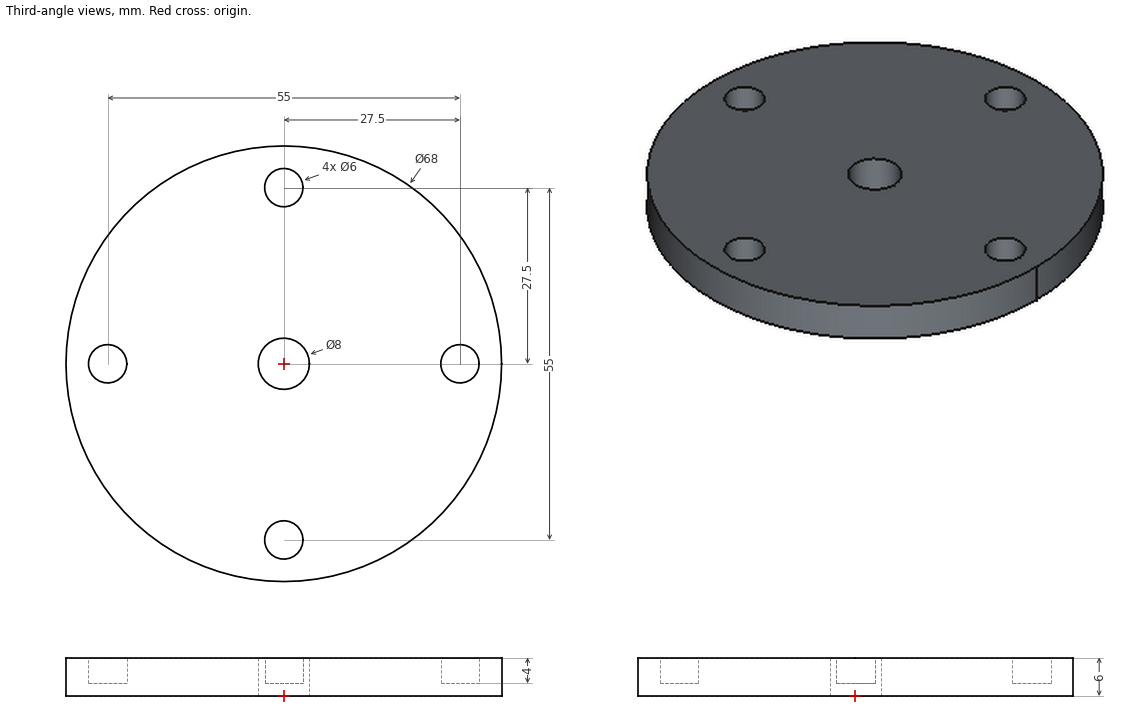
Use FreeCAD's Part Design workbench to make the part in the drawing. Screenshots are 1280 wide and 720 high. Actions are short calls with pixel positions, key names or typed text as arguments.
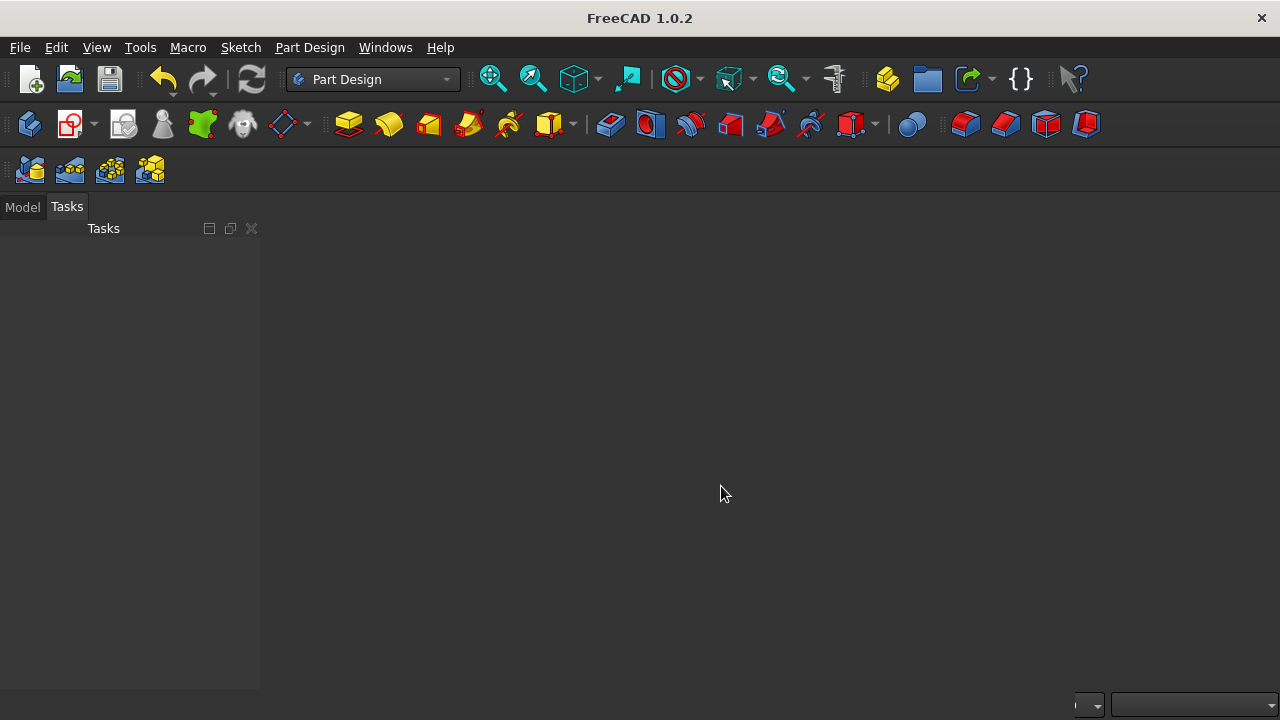
click(30, 80)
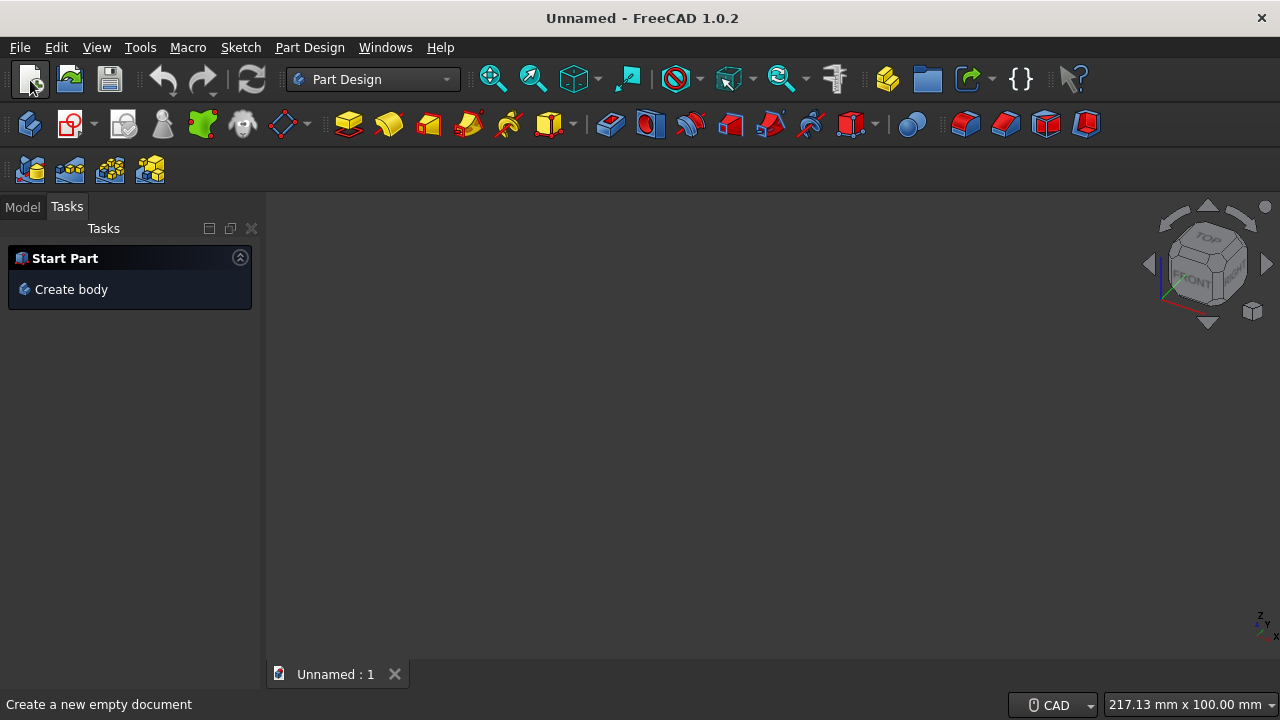
click(70, 124)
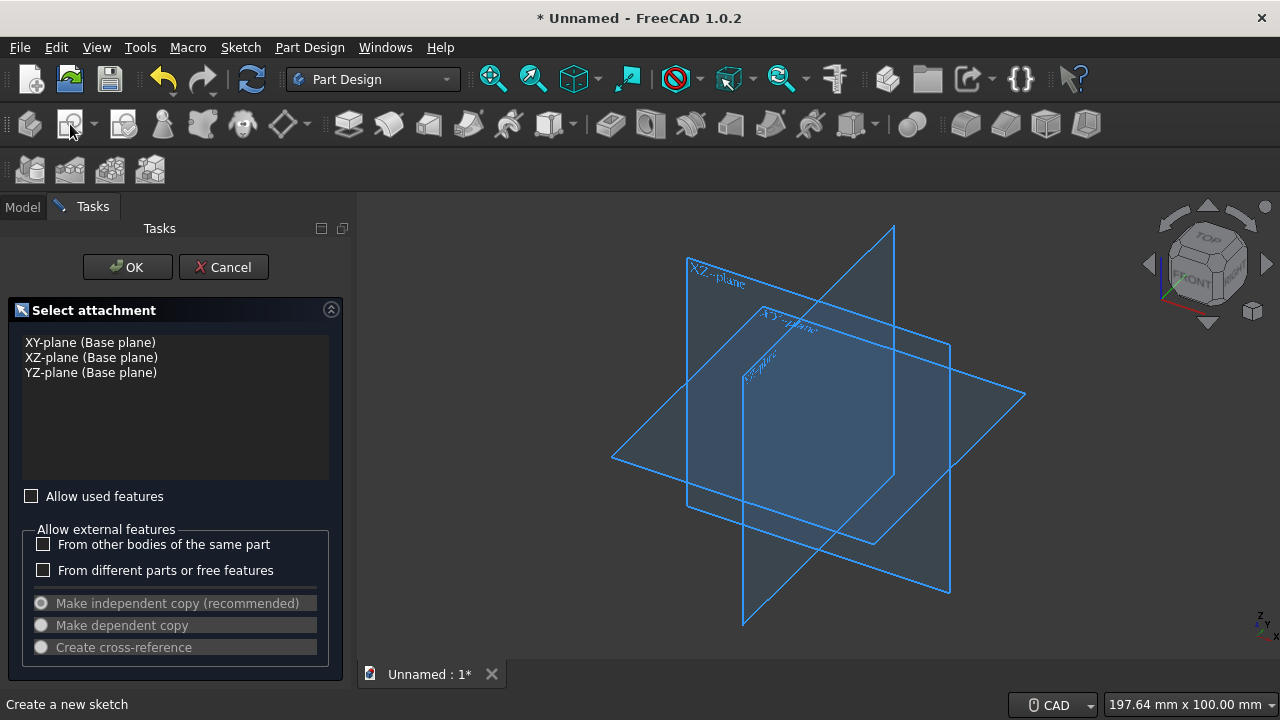
click(82, 342)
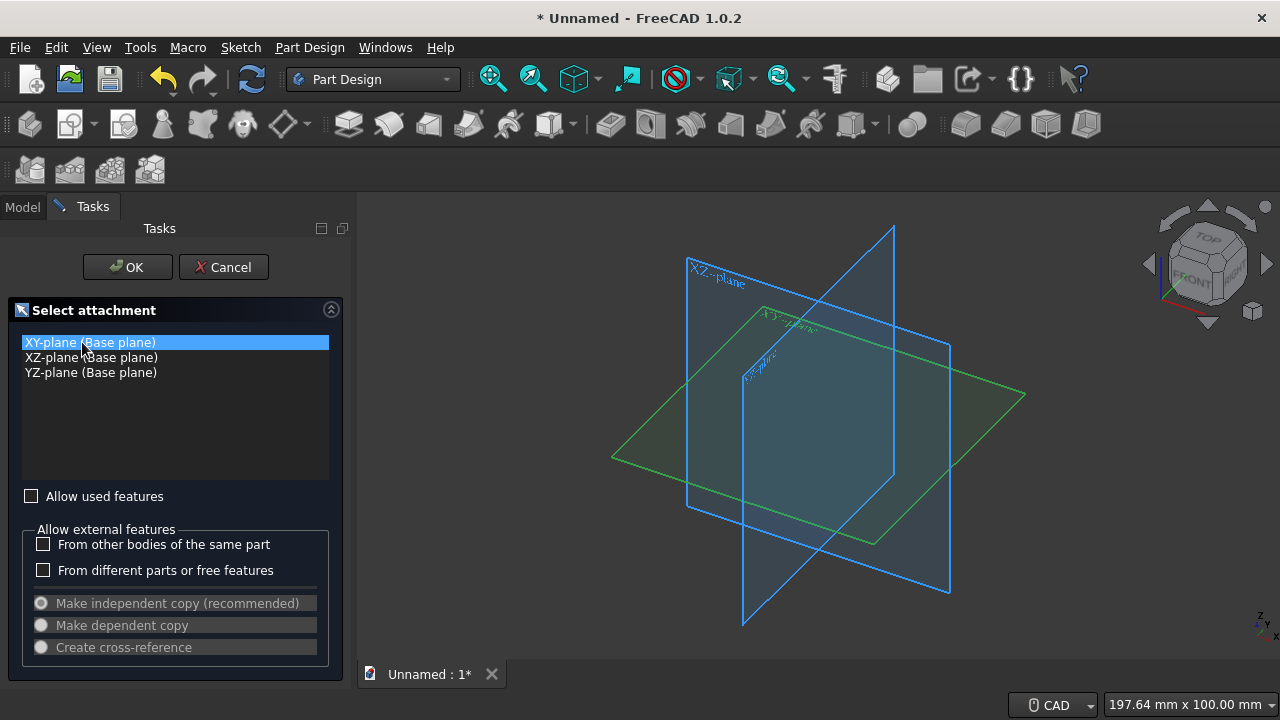
click(128, 267)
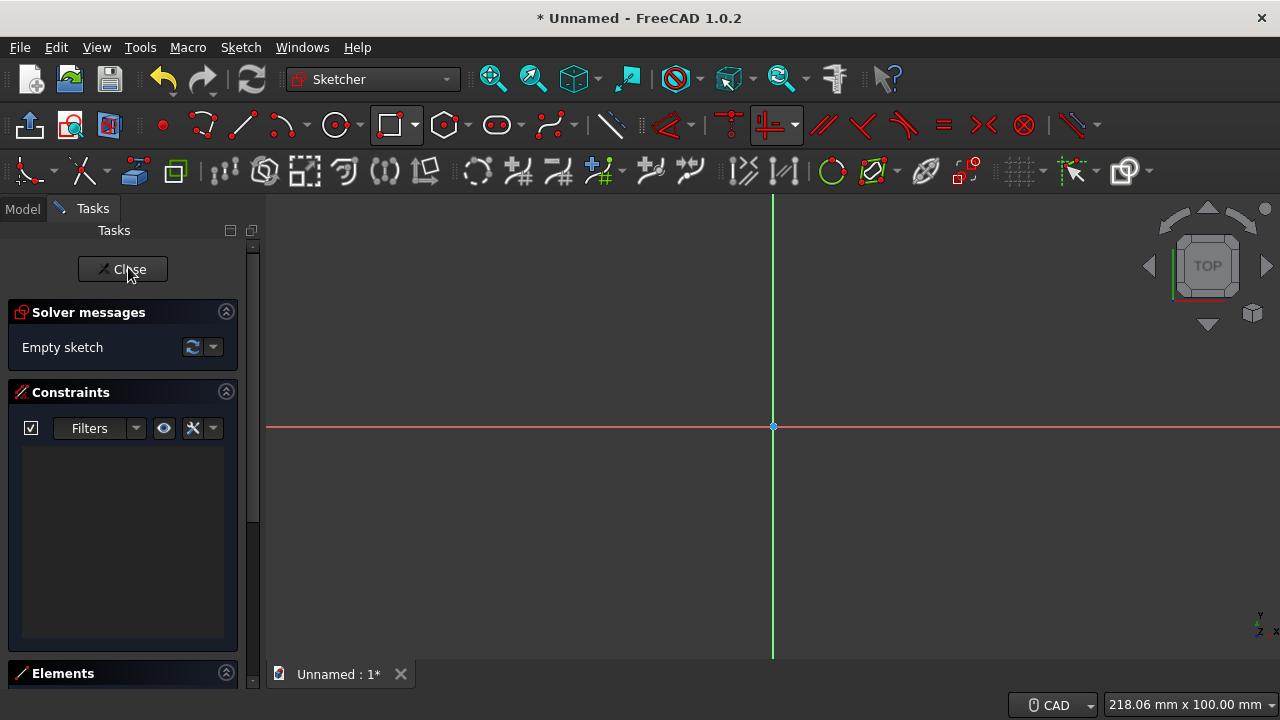
click(336, 126)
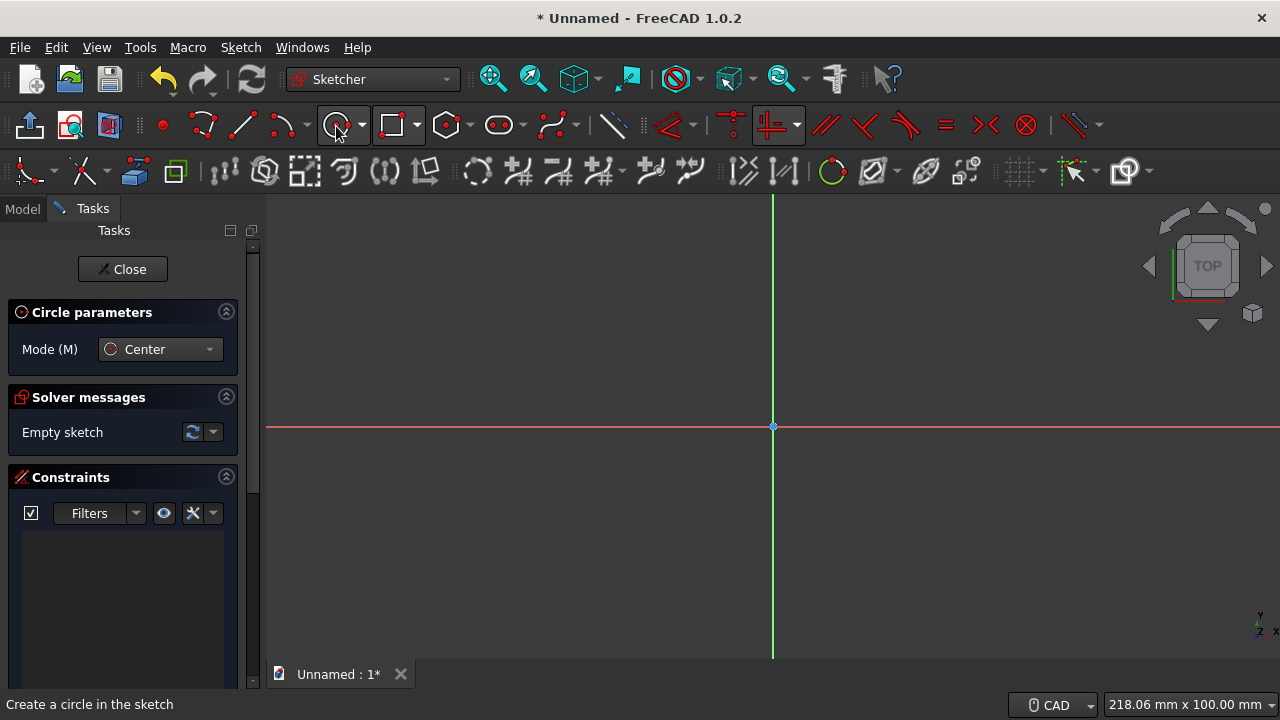
click(773, 426)
click(885, 315)
key(Escape)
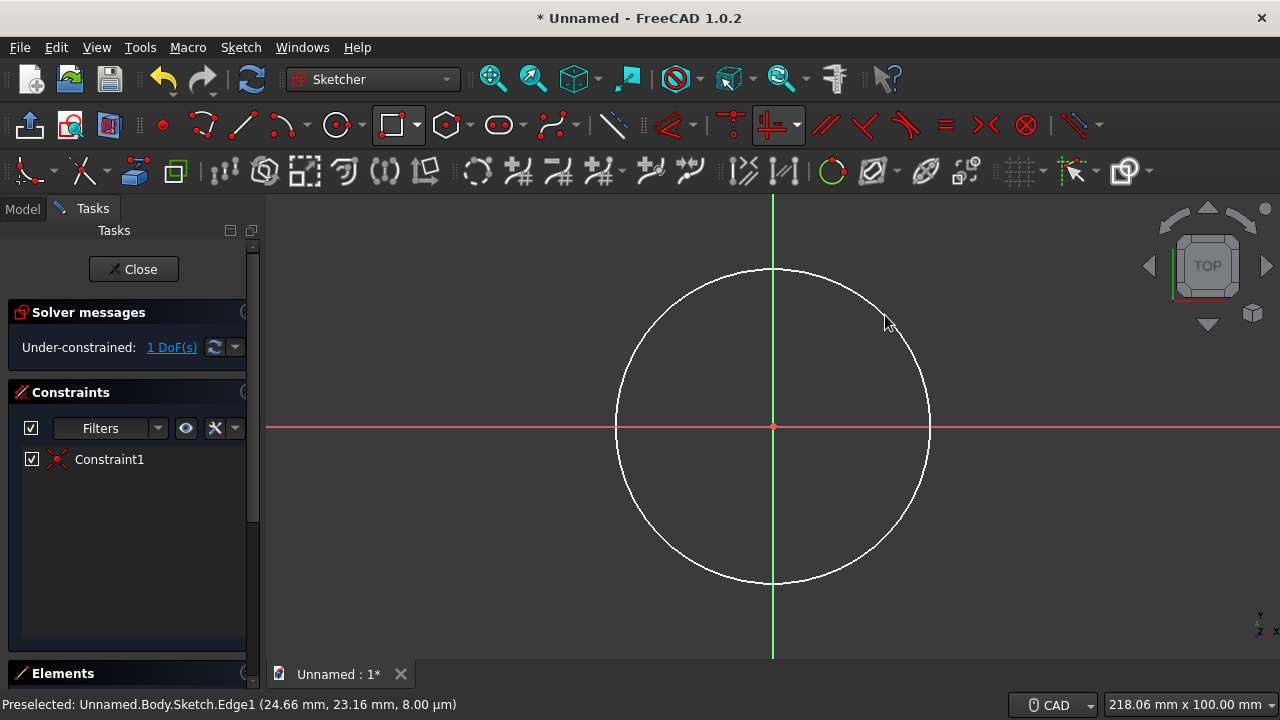
click(668, 126)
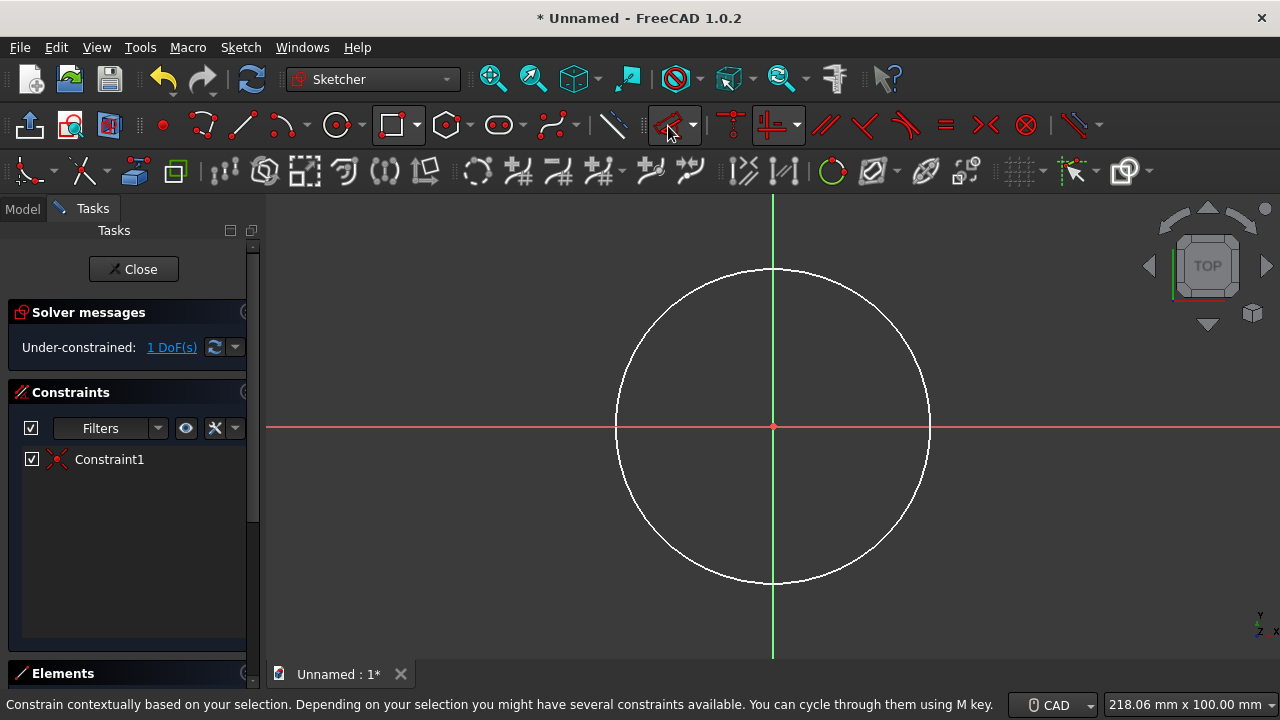
click(884, 315)
click(907, 292)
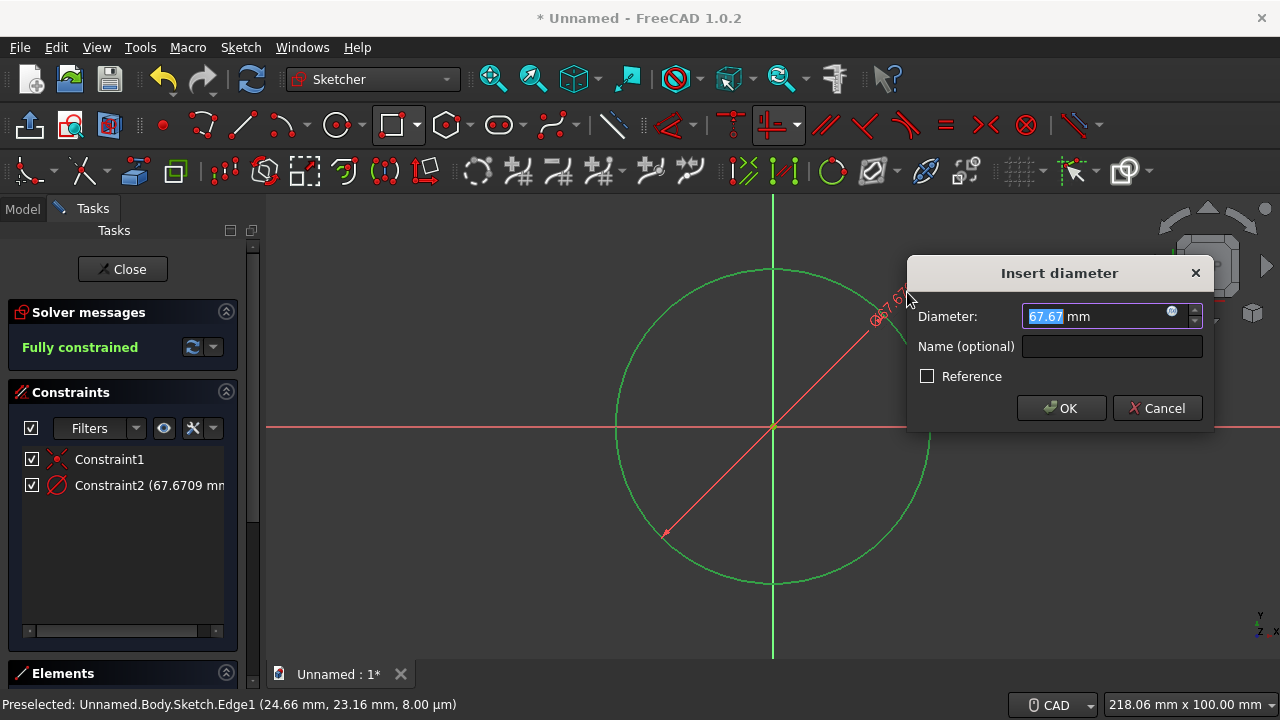
text(68)
key(Return)
key(Escape)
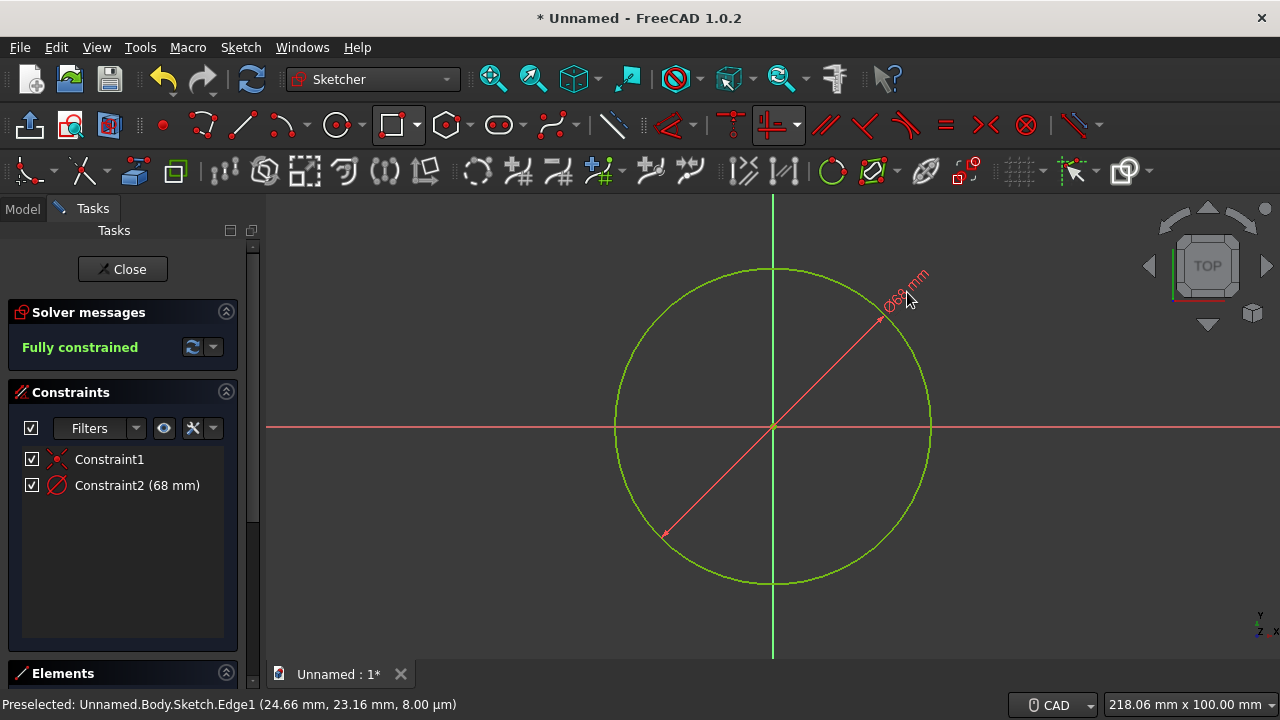
click(123, 269)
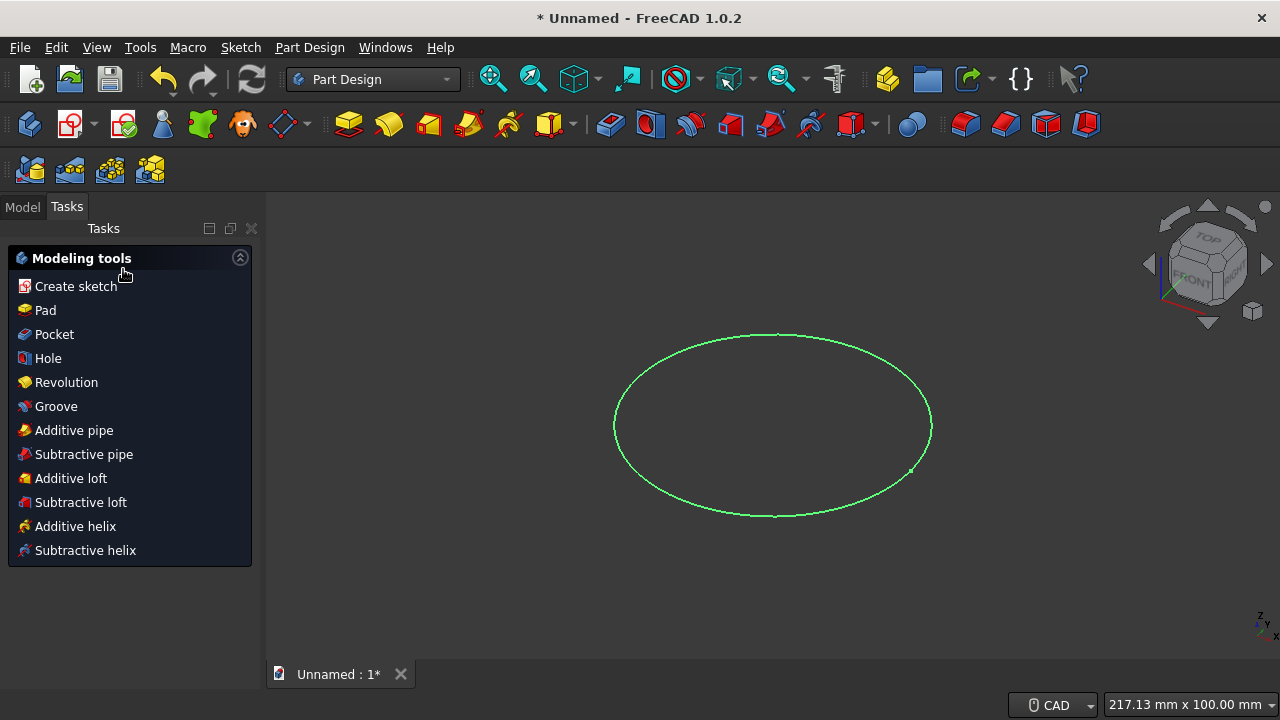
click(350, 124)